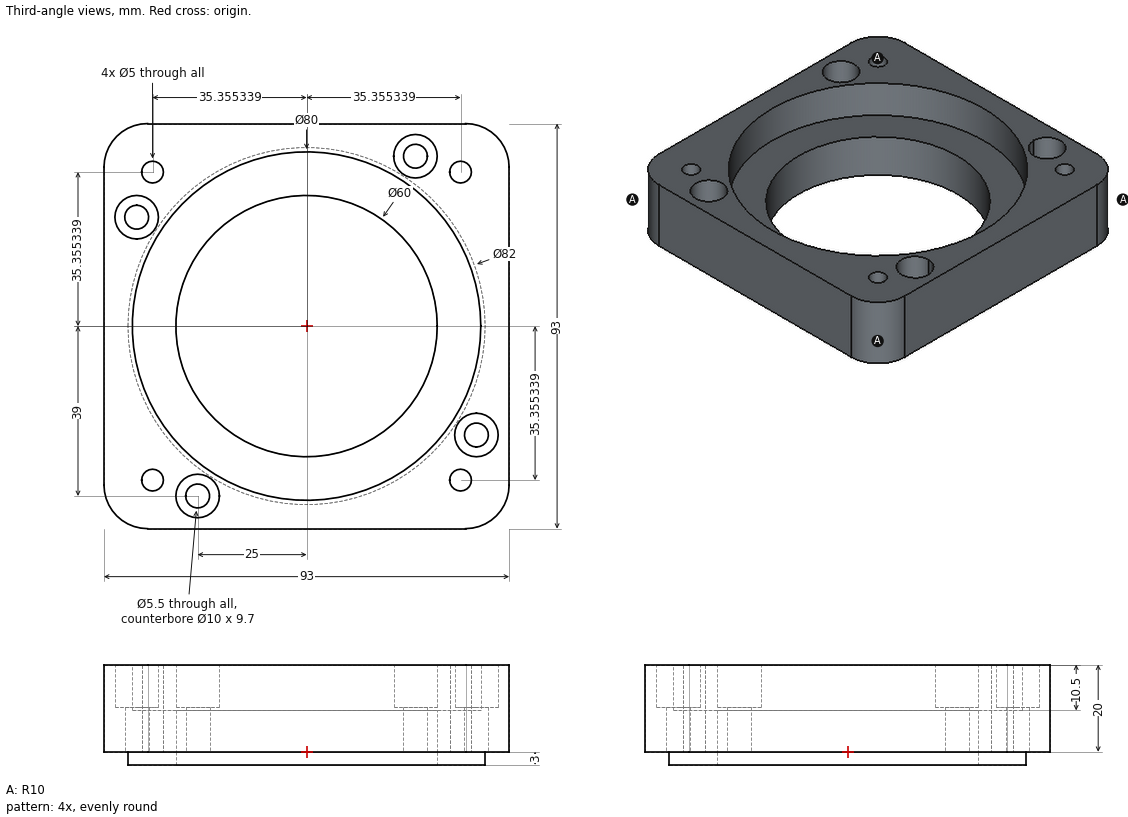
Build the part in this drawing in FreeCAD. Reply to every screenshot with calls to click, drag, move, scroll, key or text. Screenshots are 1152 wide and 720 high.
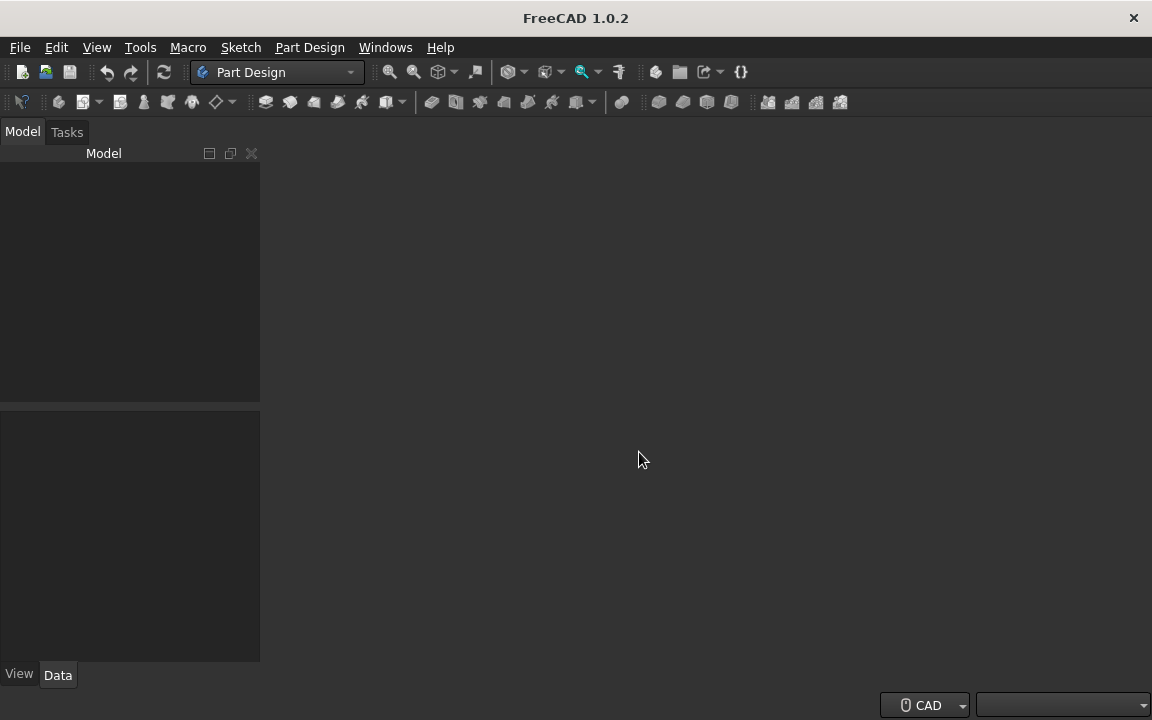
click(22, 72)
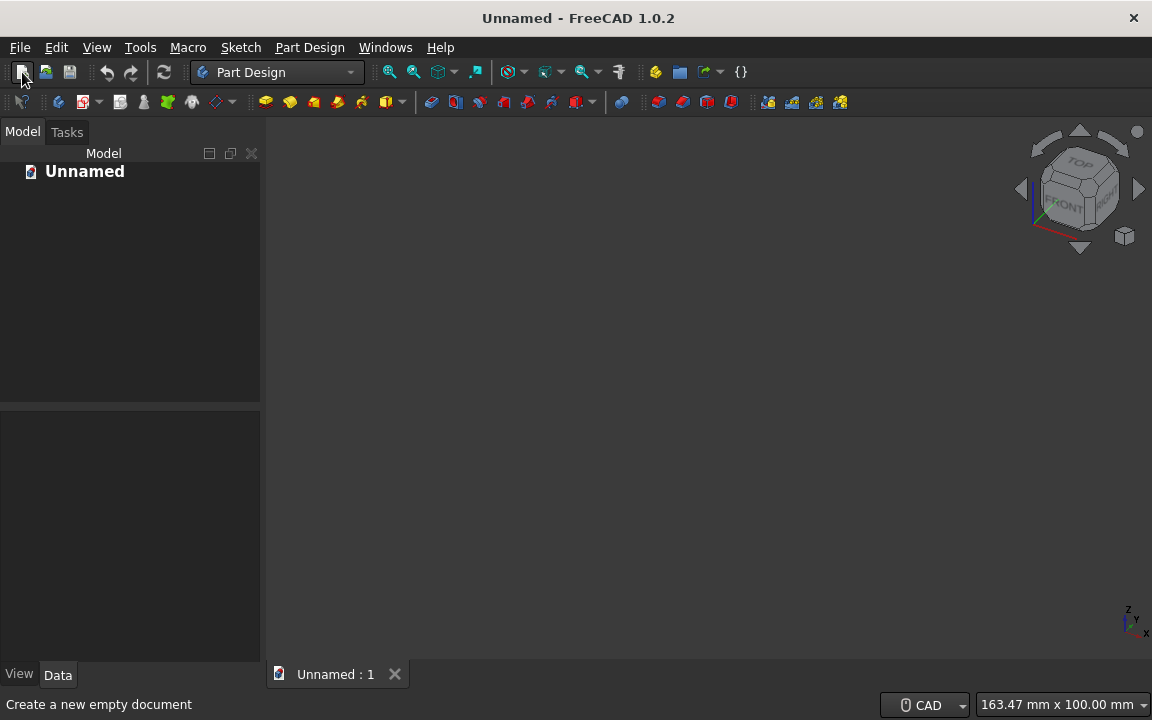
click(84, 102)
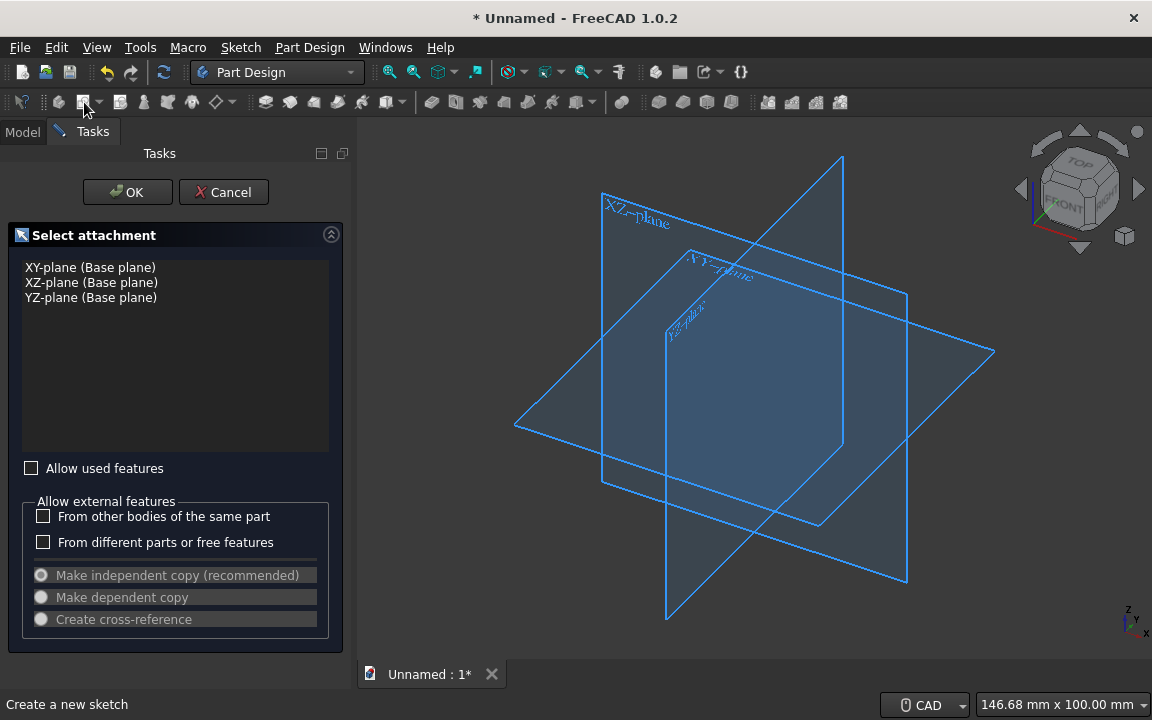
click(82, 268)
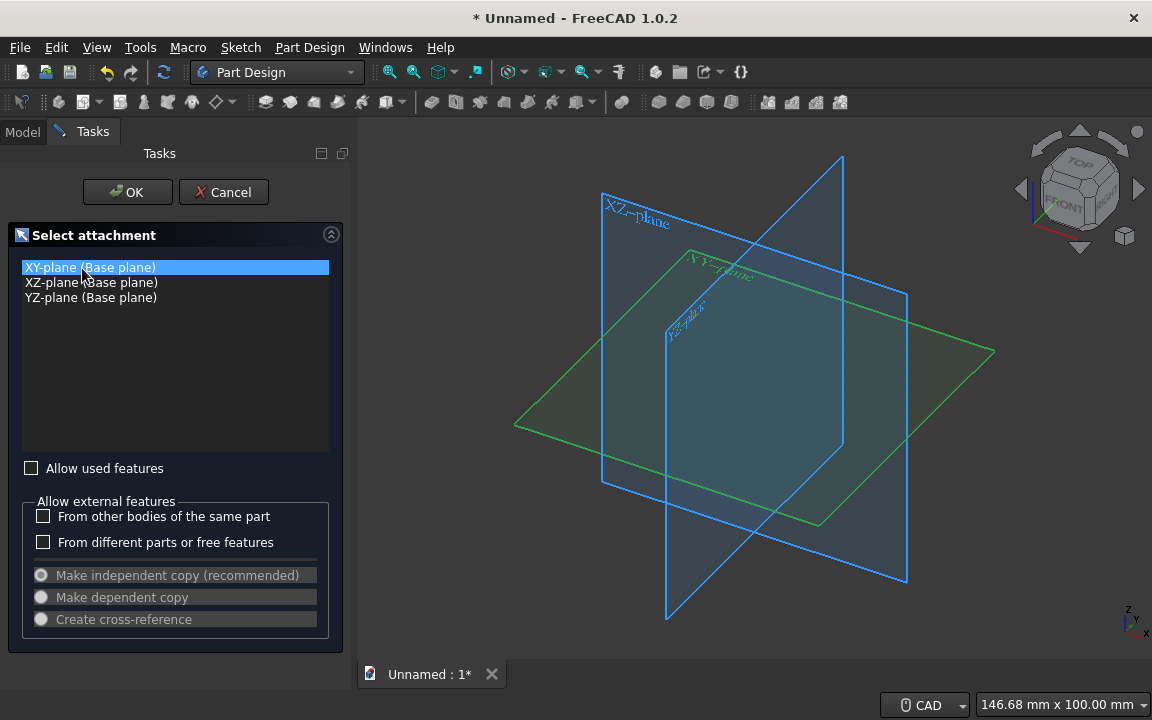
click(128, 192)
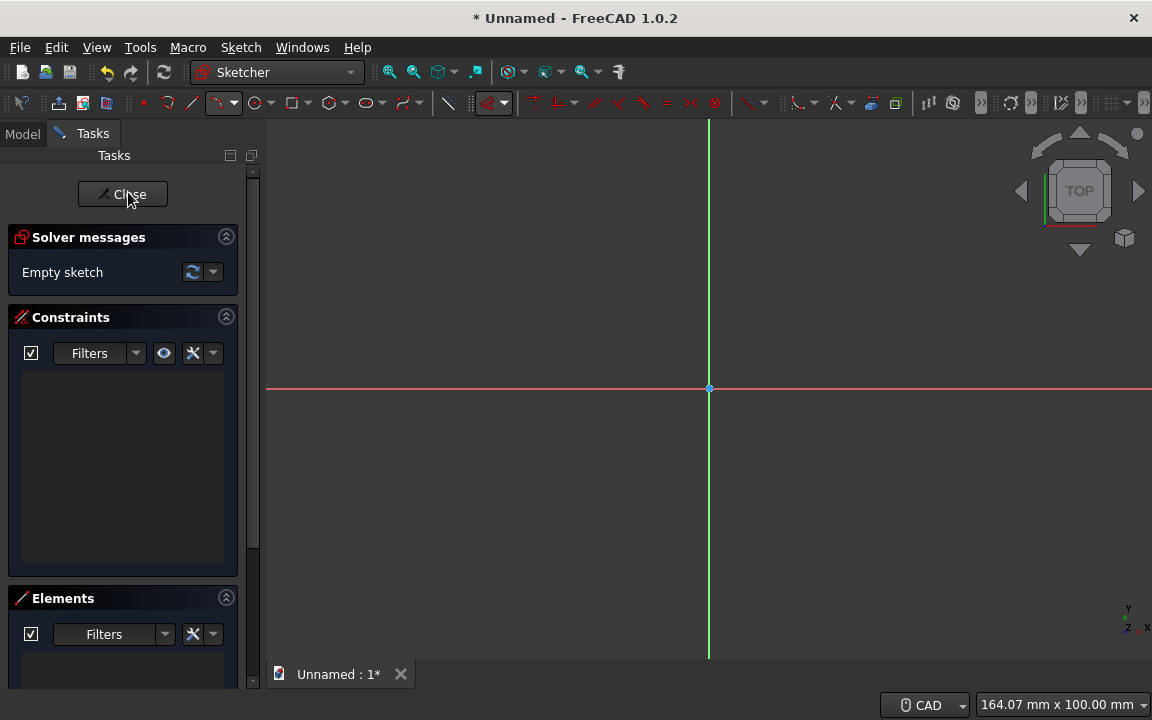
scroll(501, 389, down, 2)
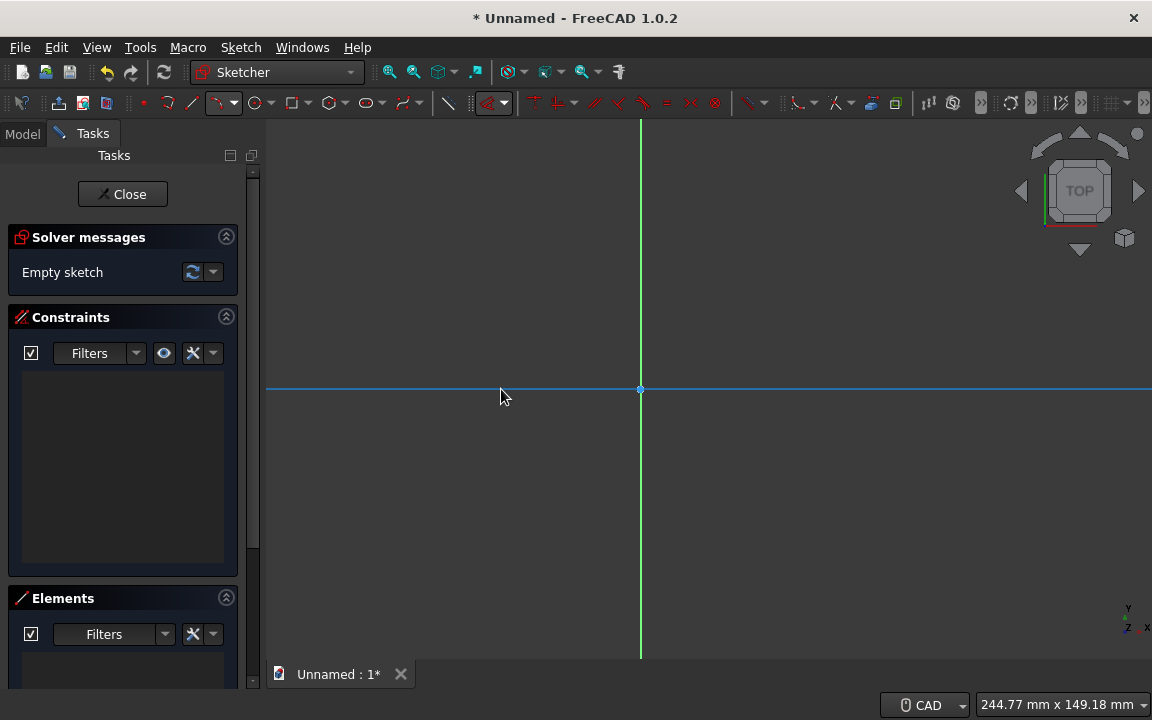
key(g)
key(v)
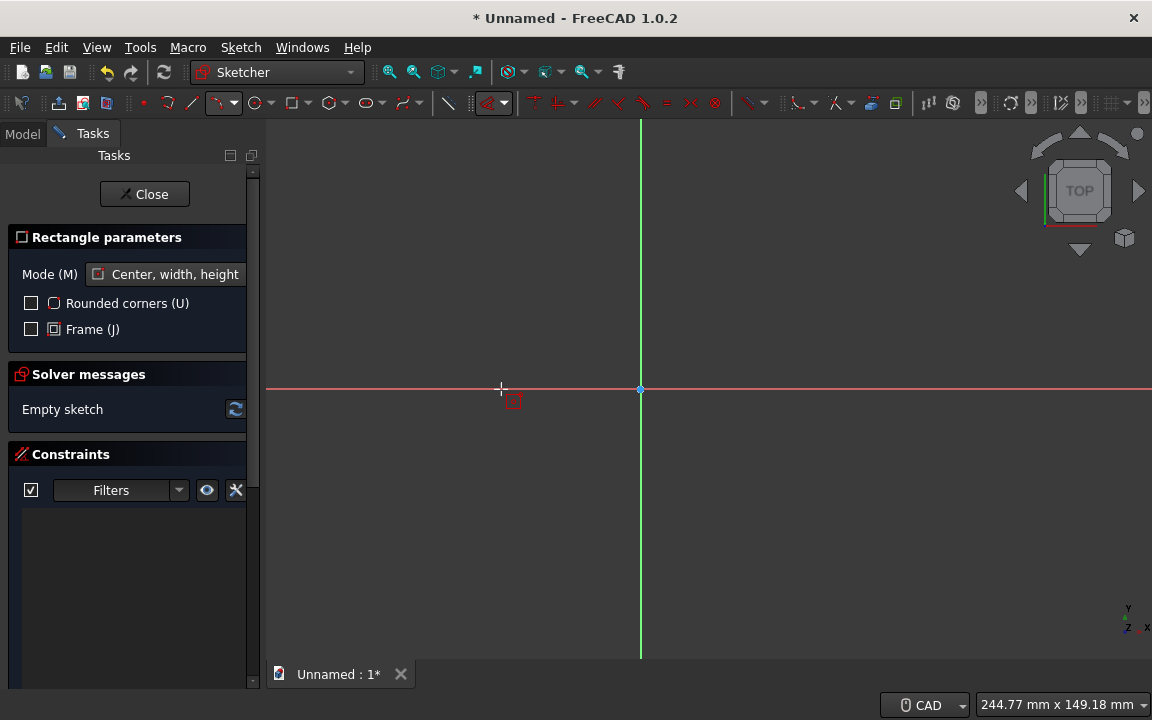
click(641, 389)
click(809, 221)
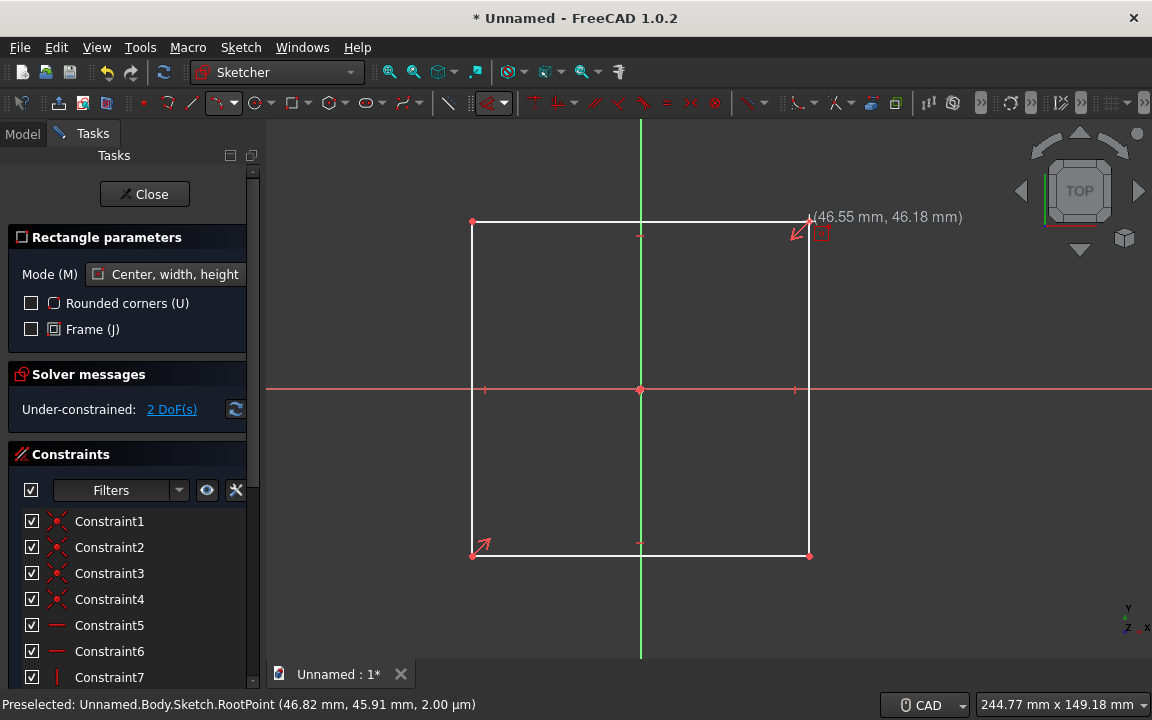
click(256, 104)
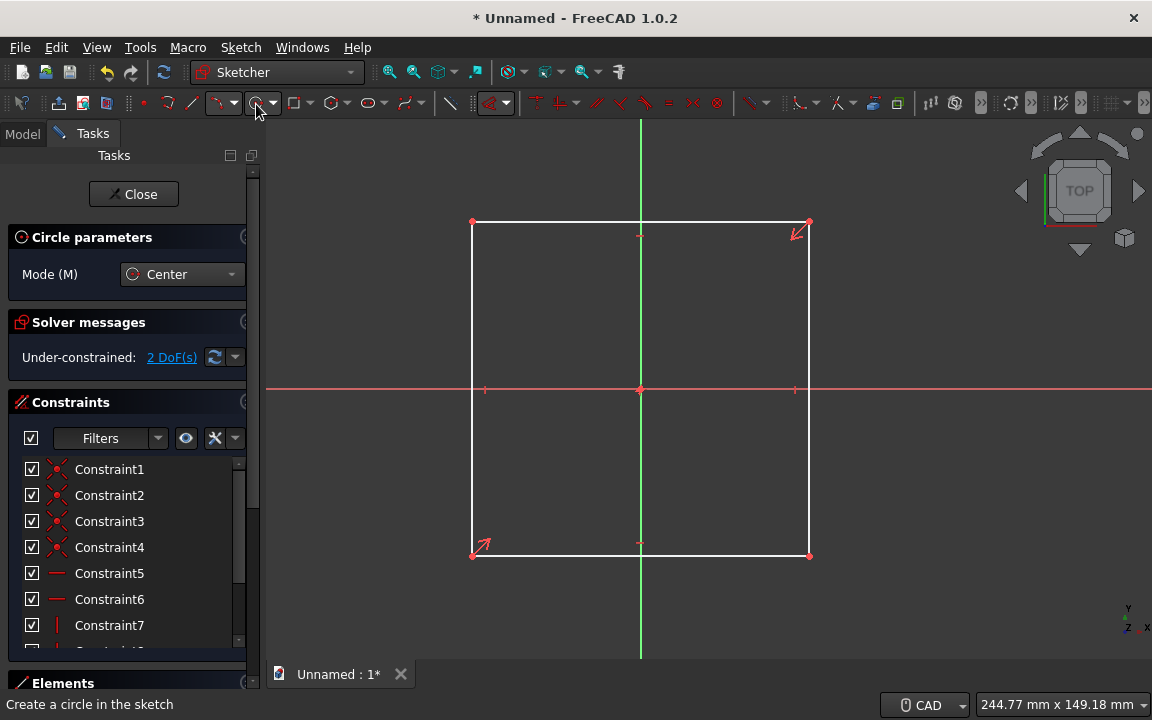
click(641, 389)
click(717, 312)
key(Escape)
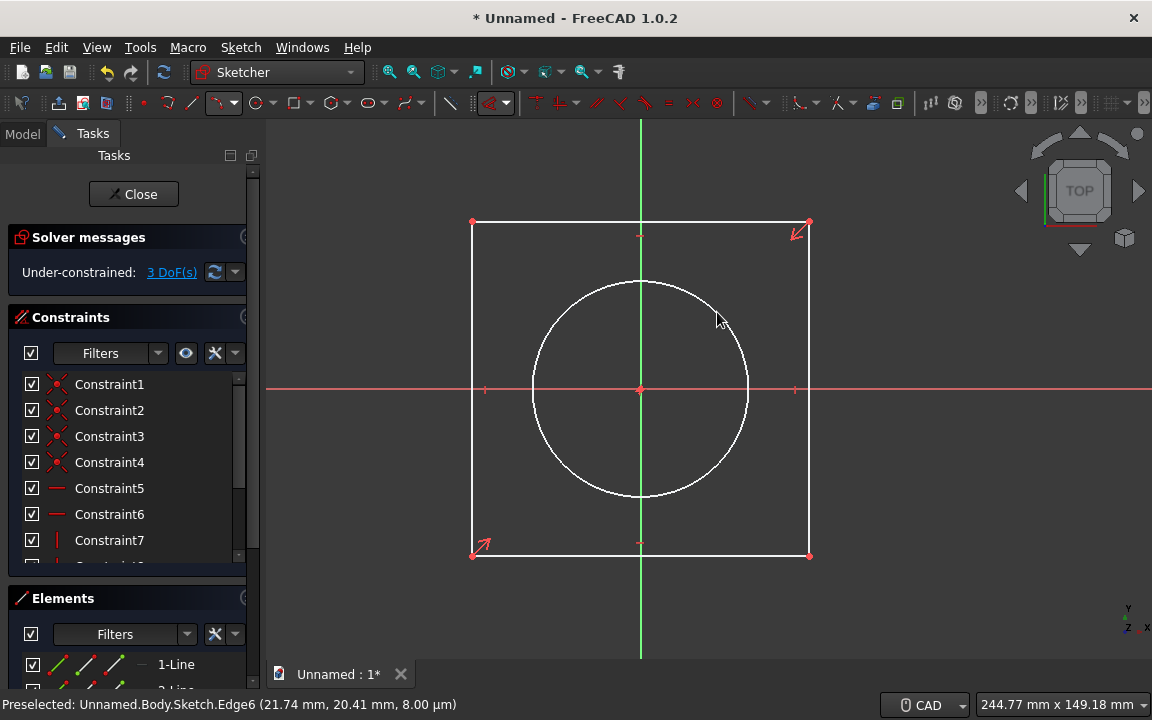
click(490, 104)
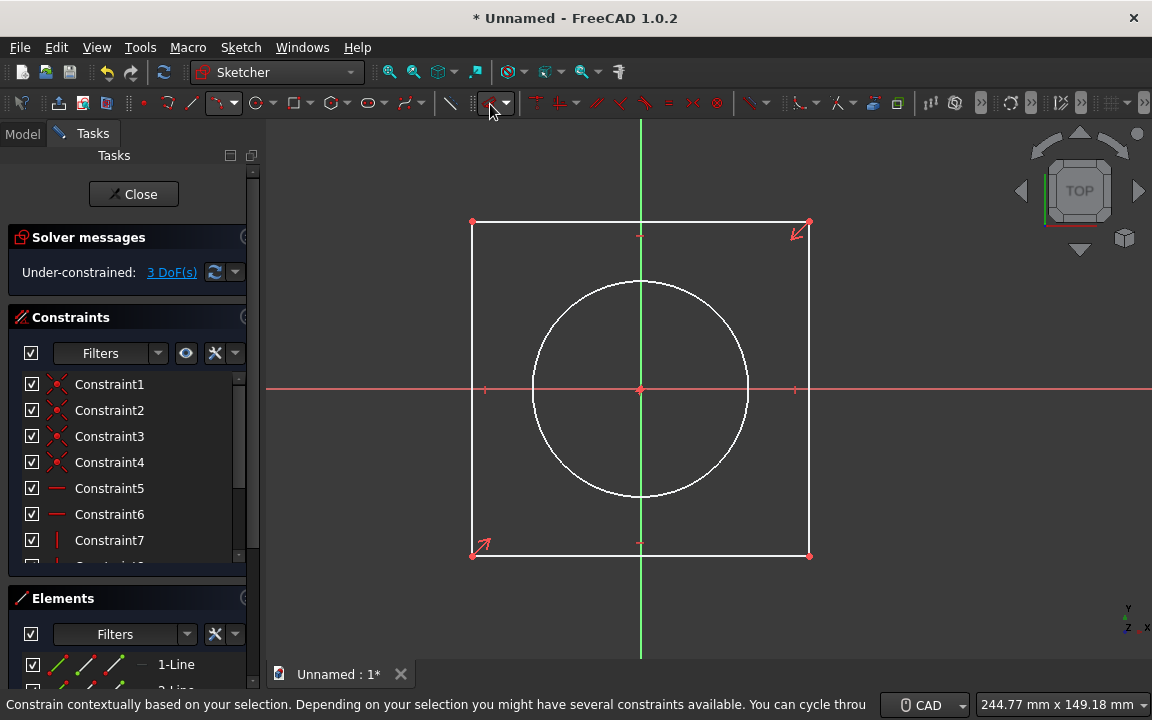
click(717, 313)
click(740, 290)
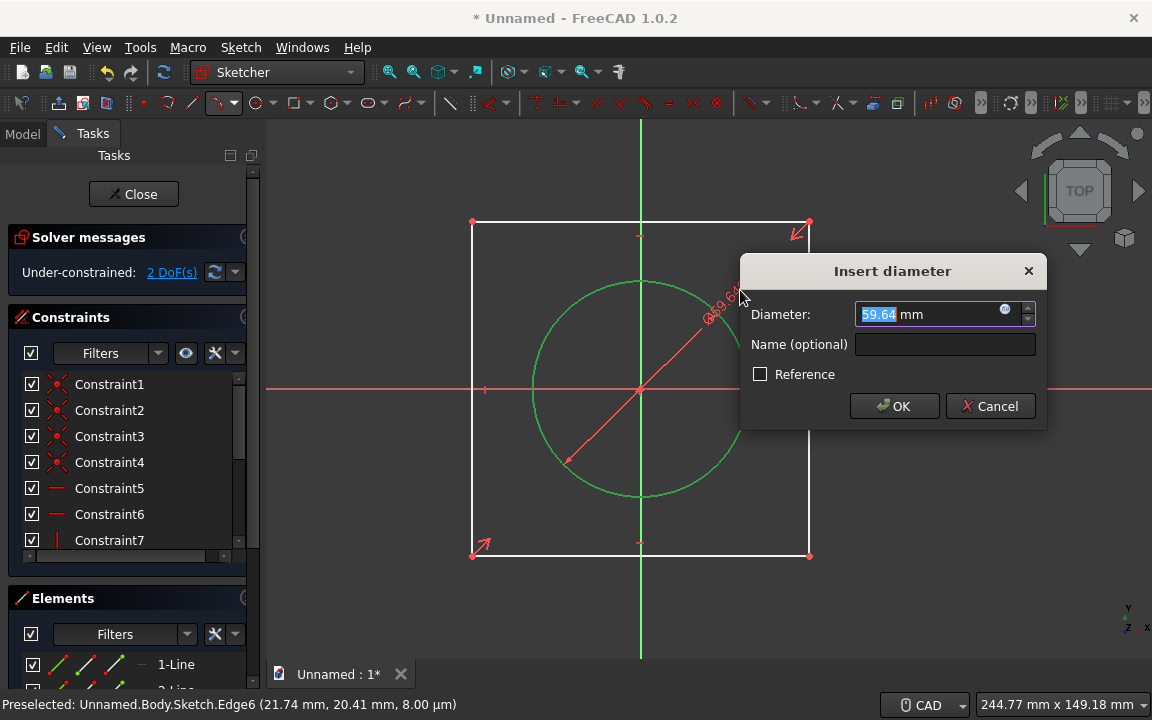
text(60)
key(Return)